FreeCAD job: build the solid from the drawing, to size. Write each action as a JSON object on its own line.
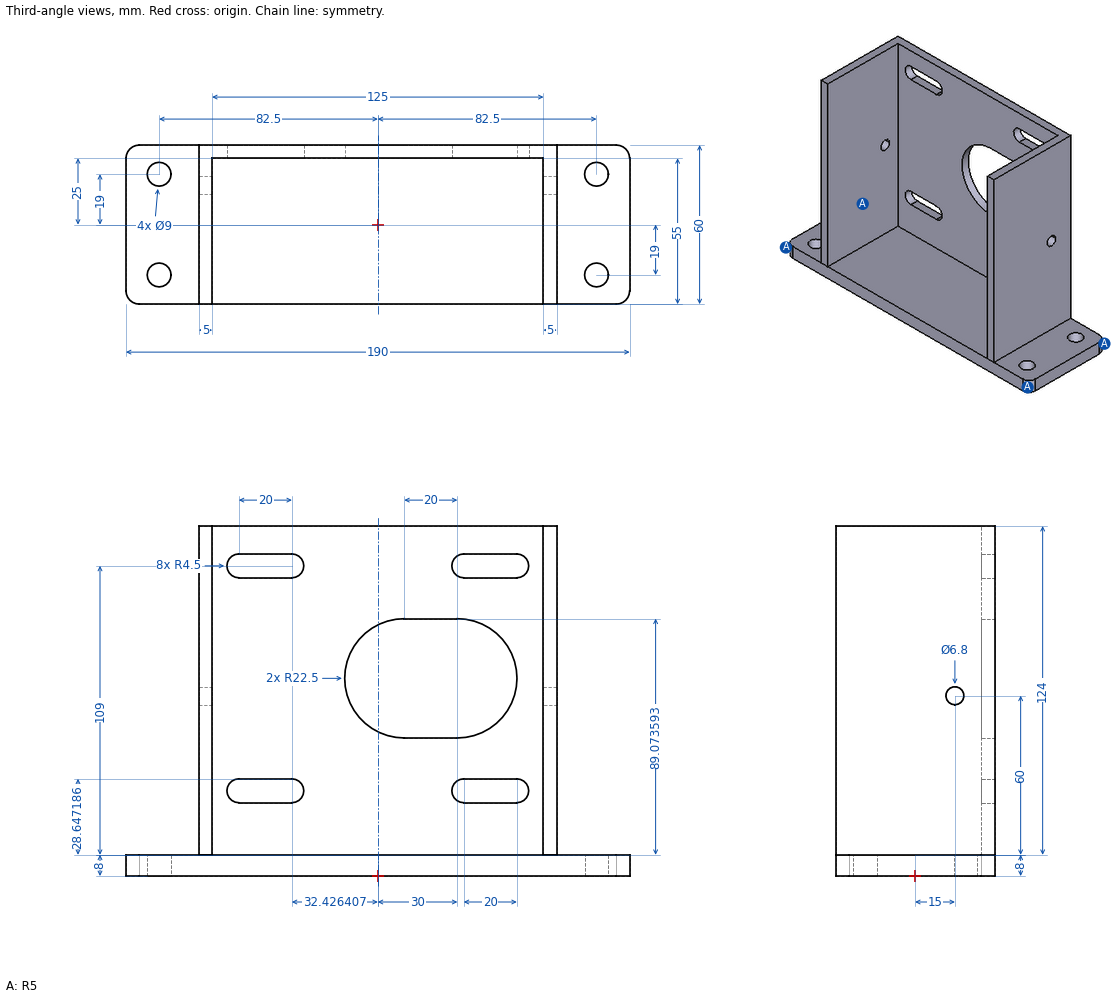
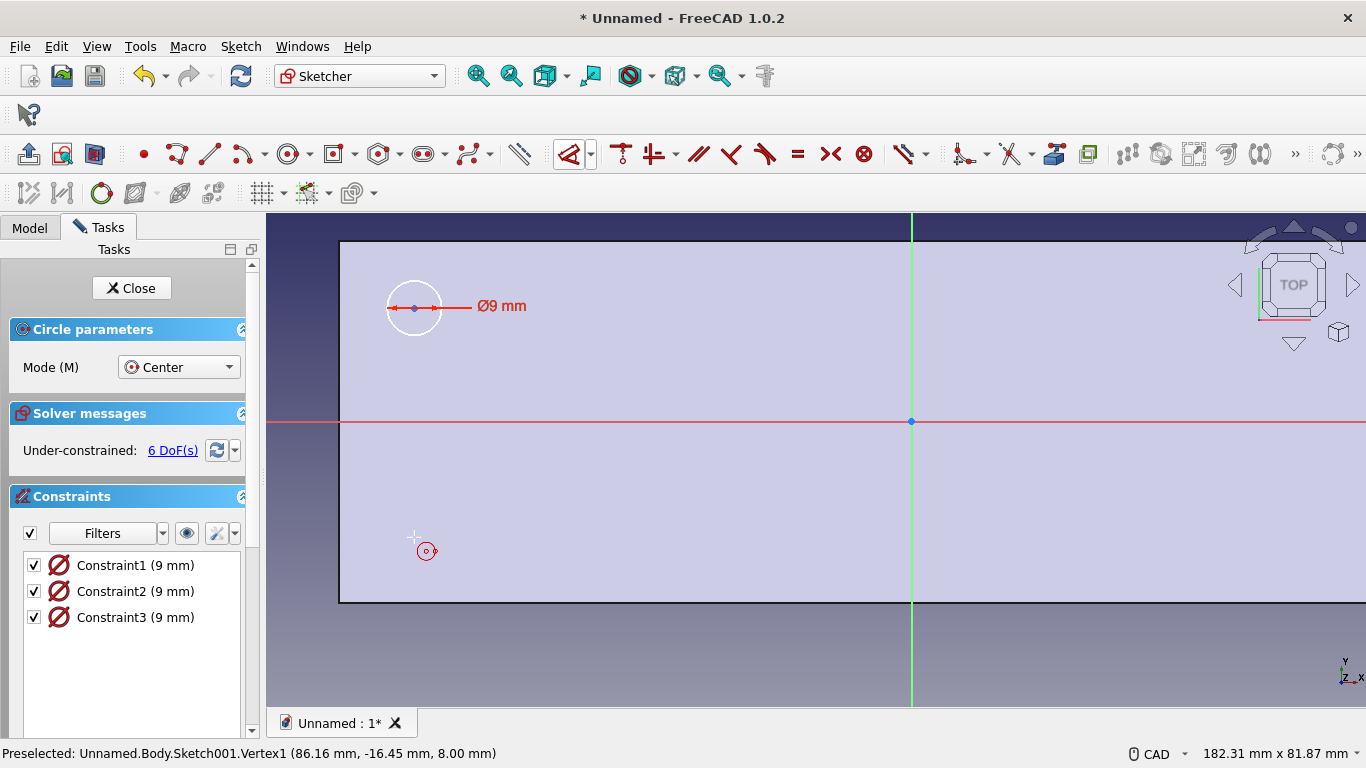
{"action": "left_click", "coordinate": [414, 537]}
{"action": "mouse_move", "coordinate": [433, 517]}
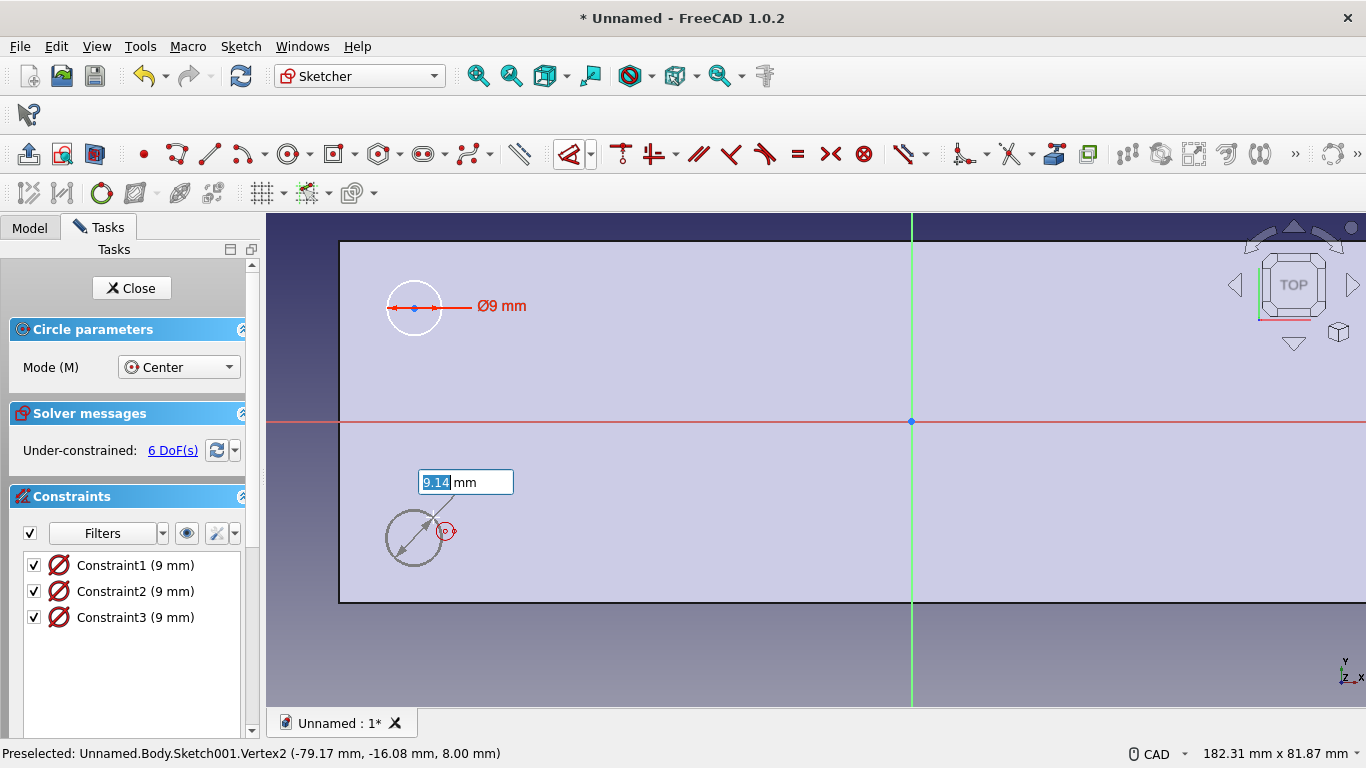
{"action": "type", "text": "9"}
{"action": "key", "text": "Return"}
{"action": "key", "text": "Escape"}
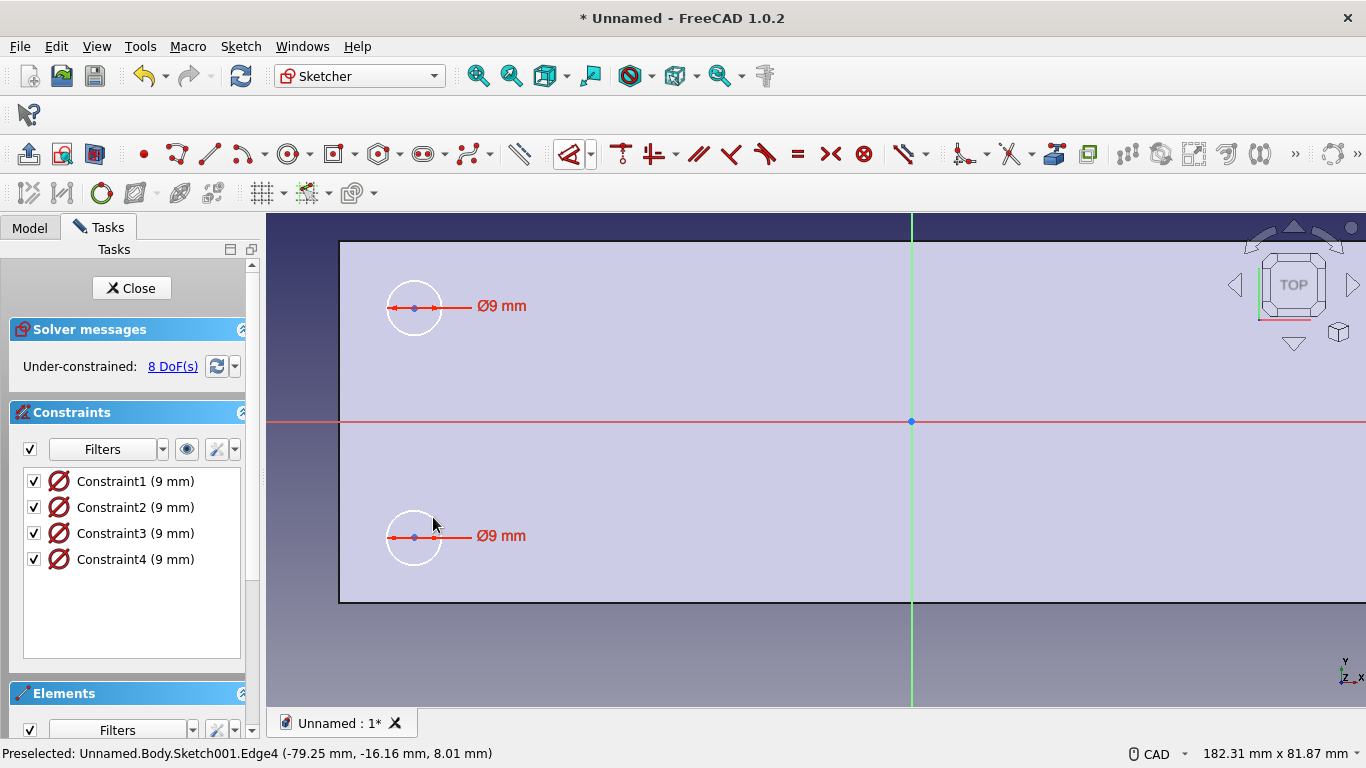
{"action": "left_click", "coordinate": [414, 308]}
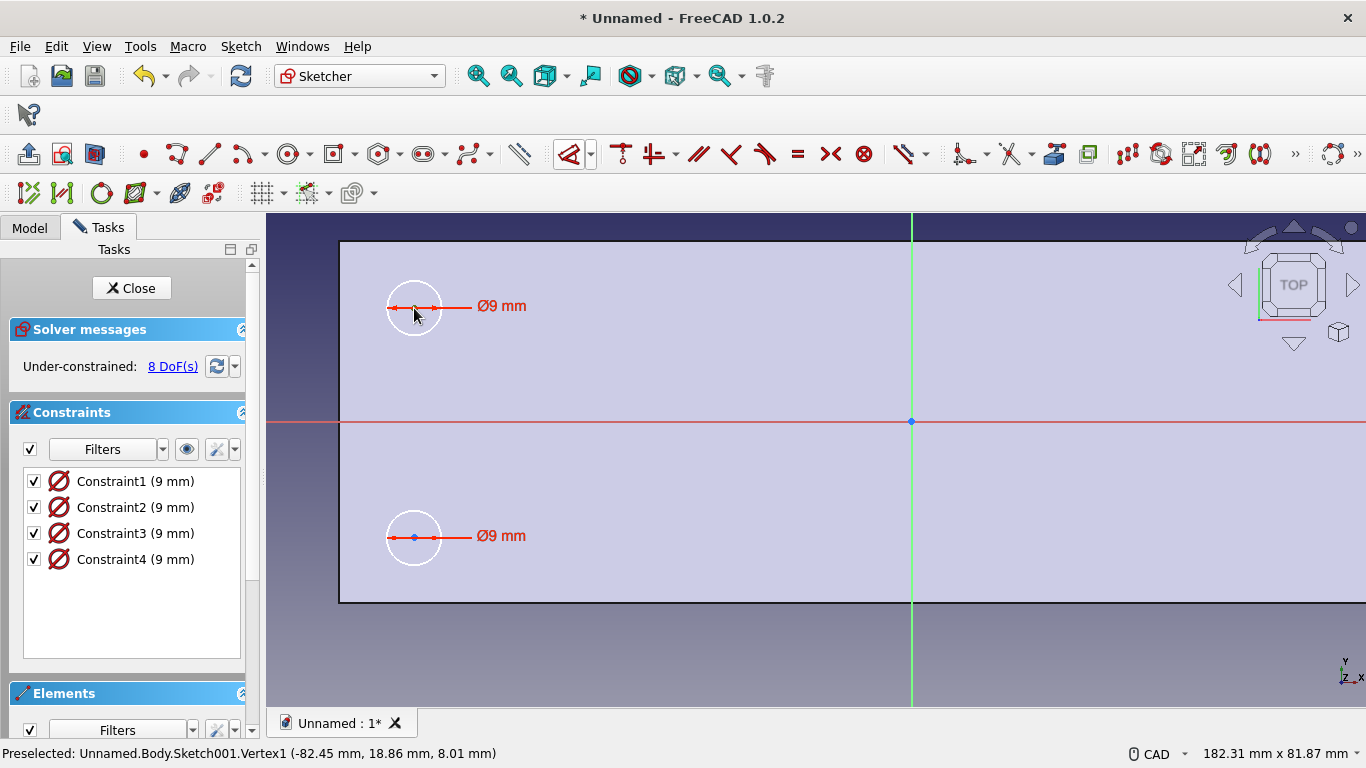
{"action": "scroll", "coordinate": [413, 537], "scroll_direction": "down", "scroll_amount": 2}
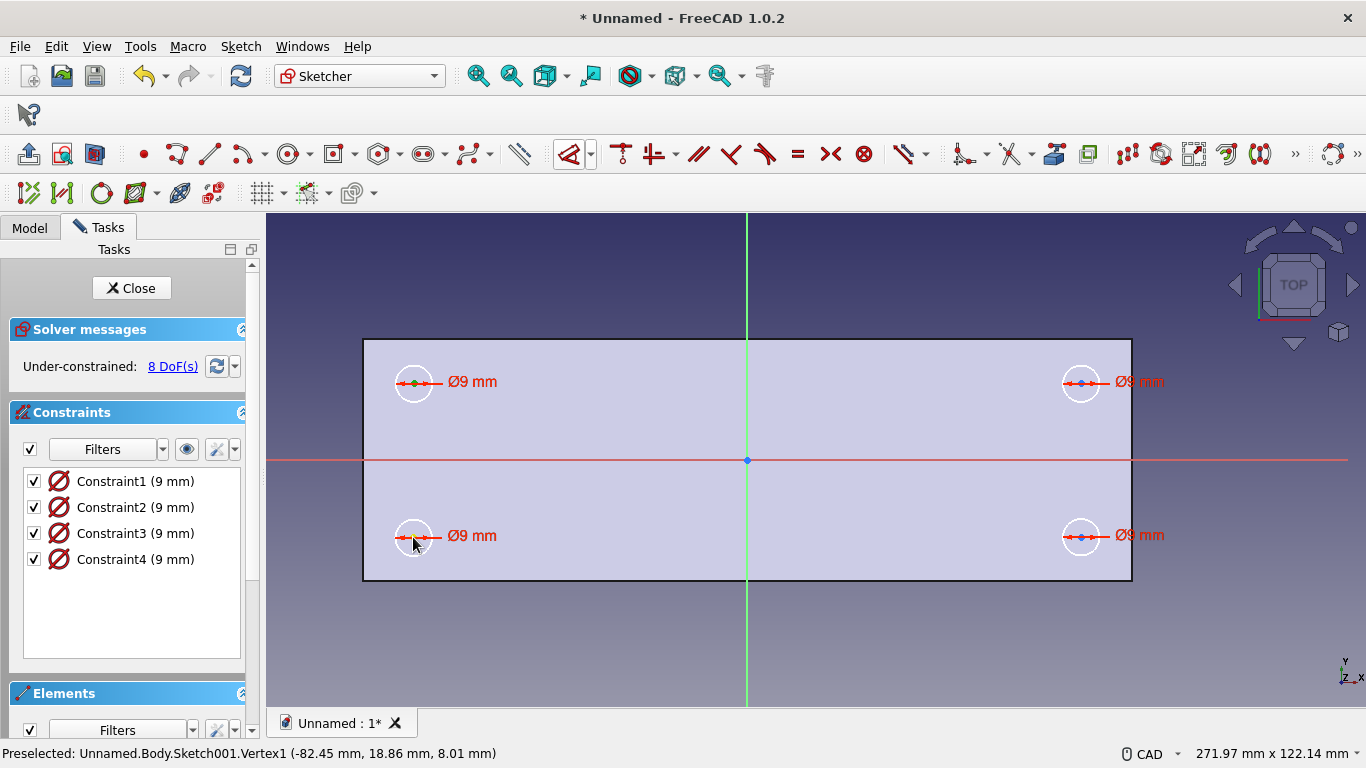
{"action": "left_click", "coordinate": [1081, 384]}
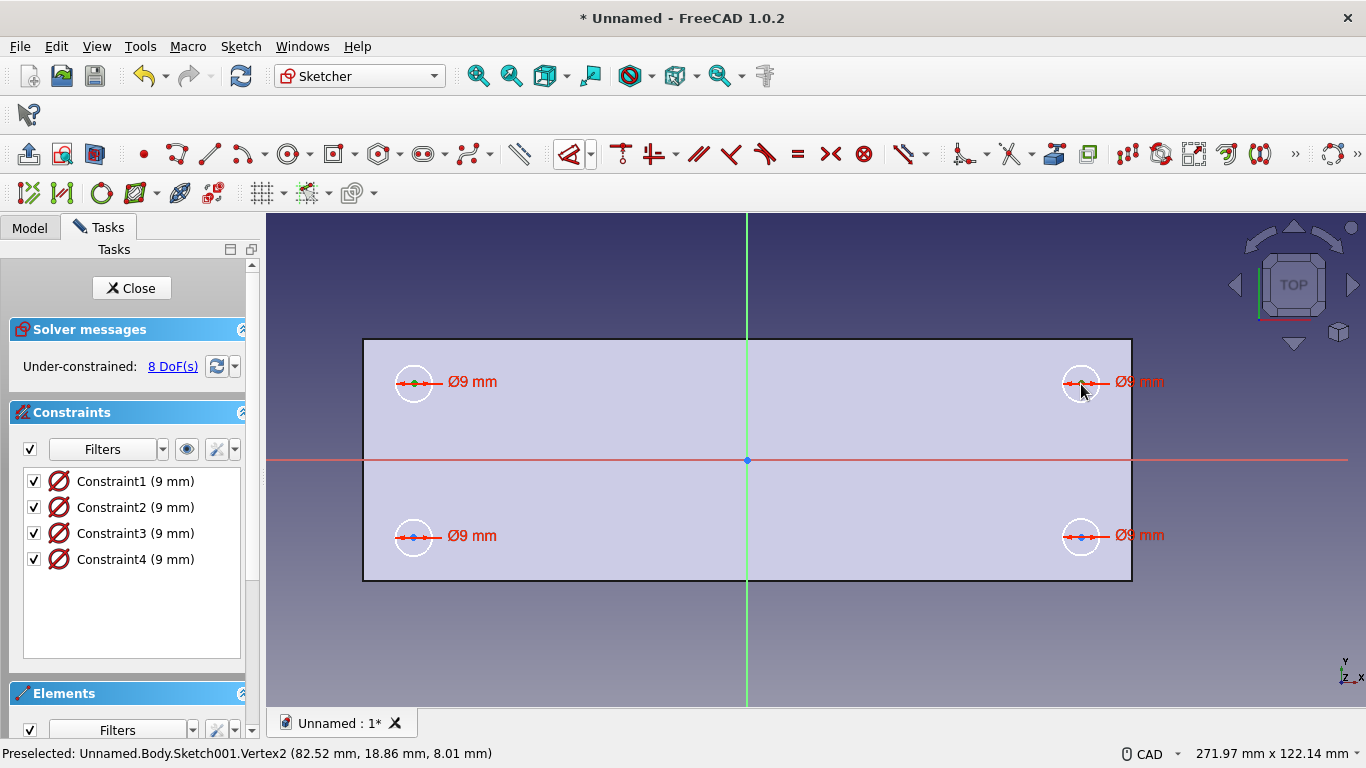
{"action": "key", "text": "h"}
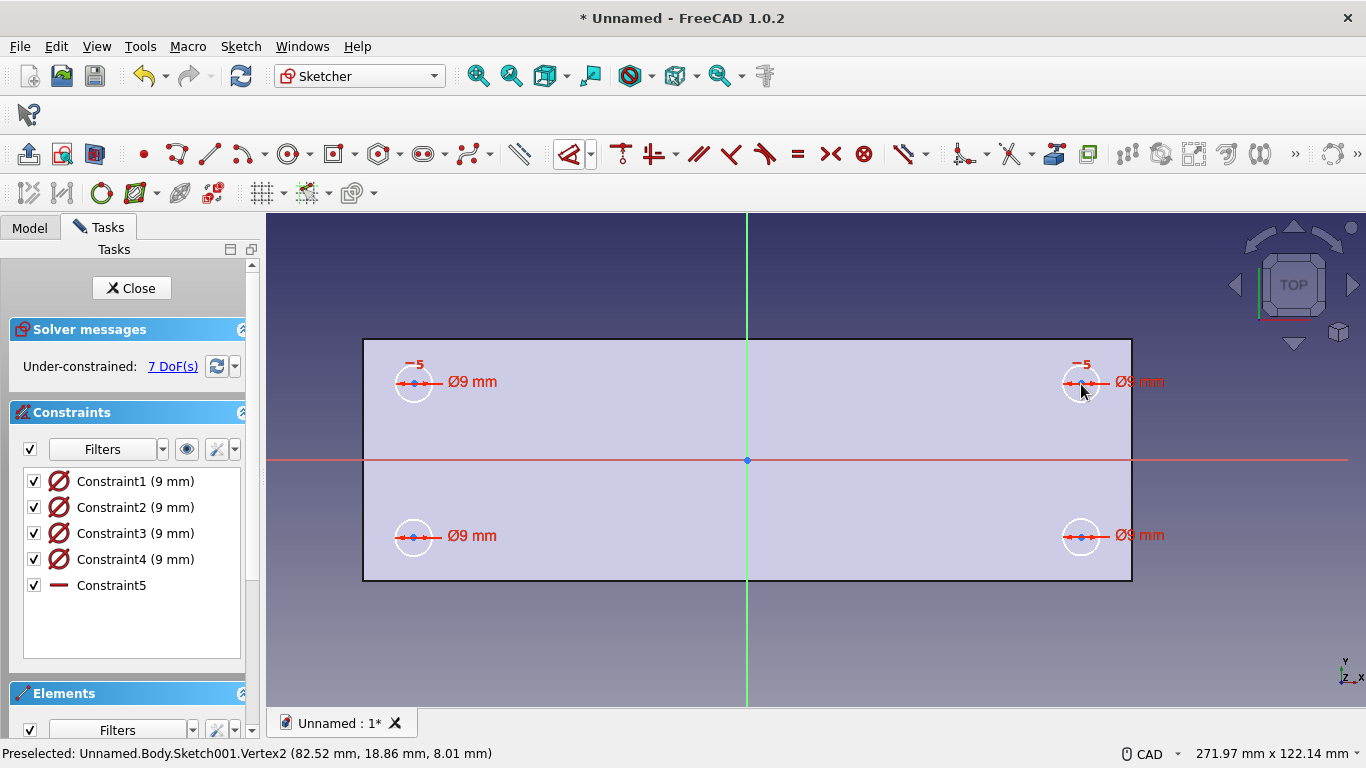
{"action": "left_click", "coordinate": [1081, 384]}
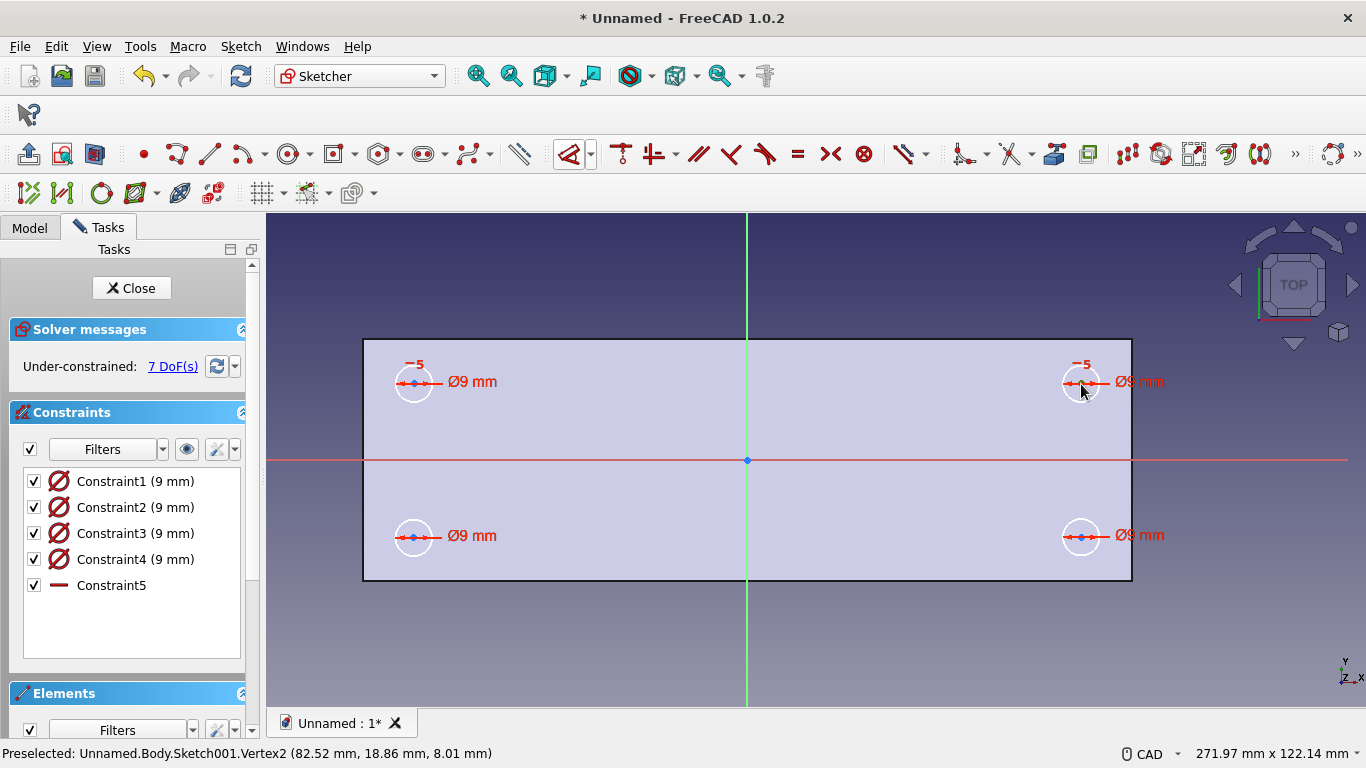
{"action": "left_click", "coordinate": [1081, 537]}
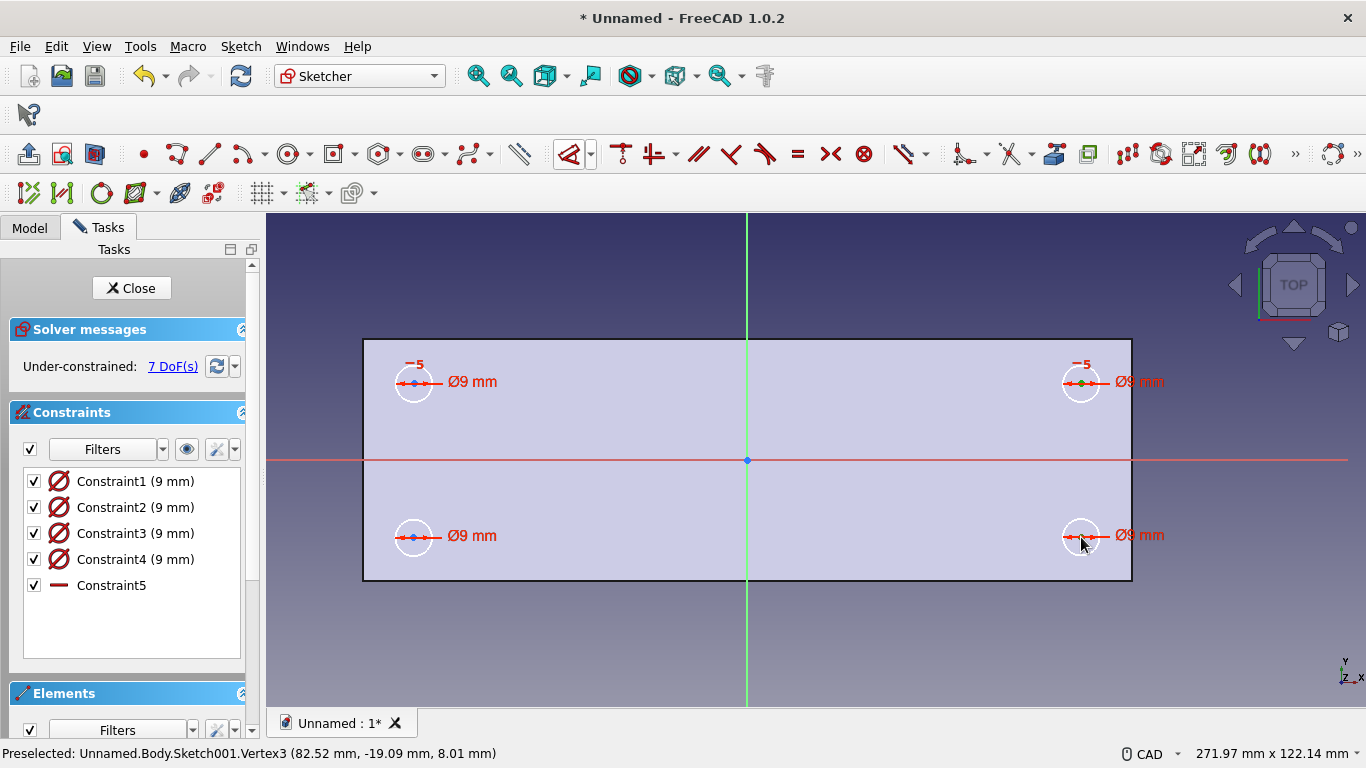
{"action": "left_click", "coordinate": [676, 154]}